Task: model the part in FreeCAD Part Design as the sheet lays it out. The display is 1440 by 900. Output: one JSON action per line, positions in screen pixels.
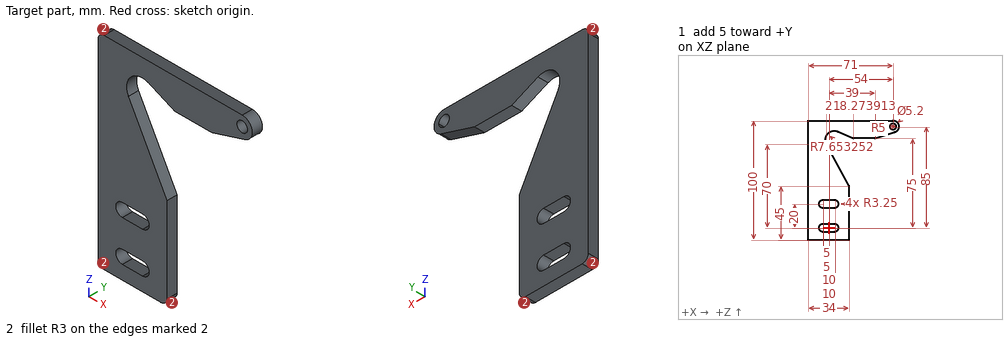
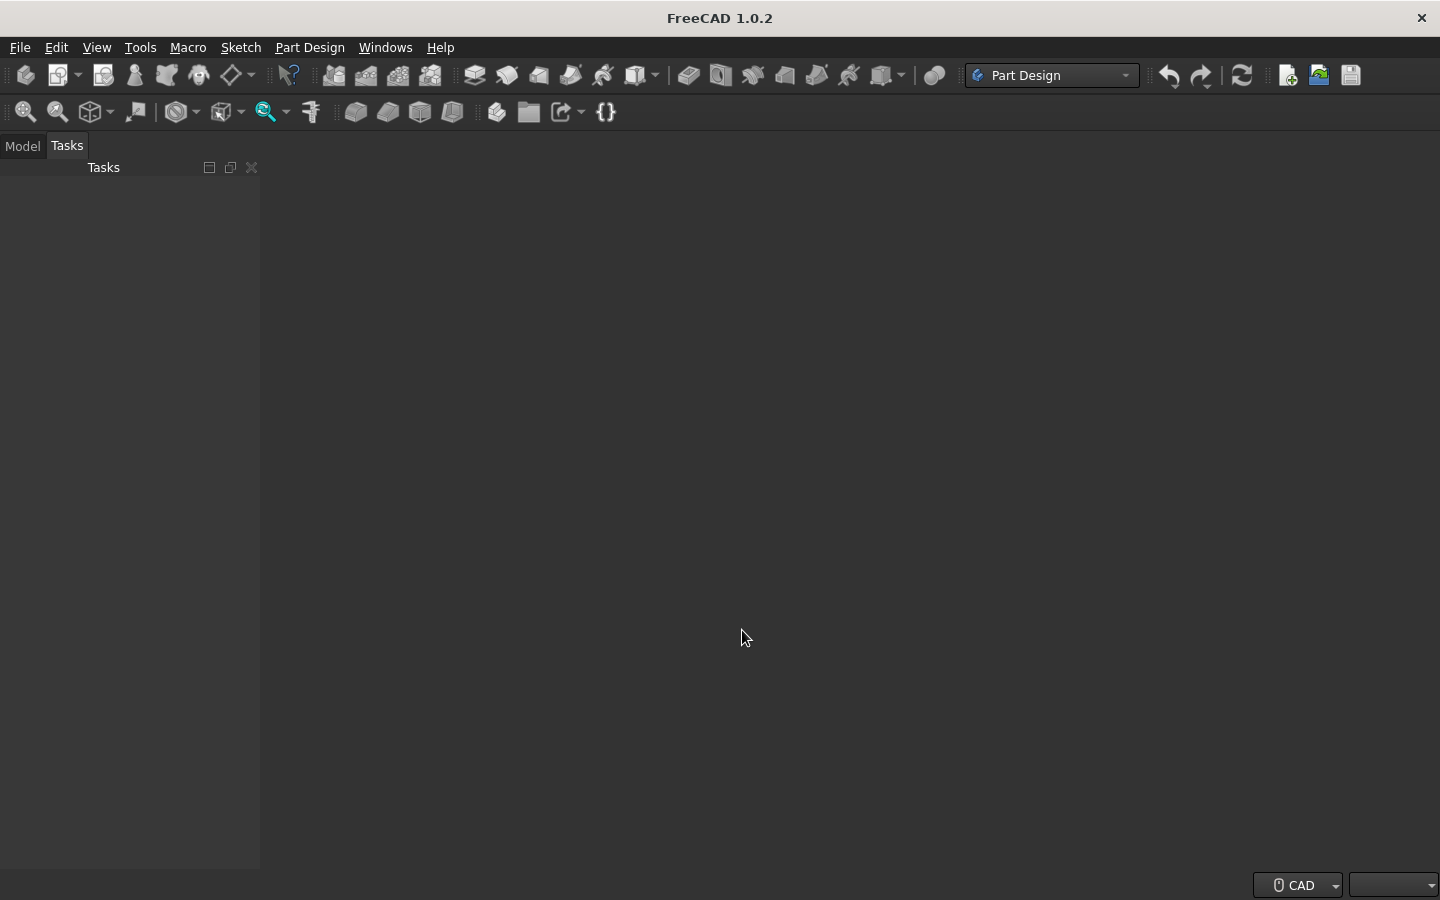
{"action": "left_click", "coordinate": [1288, 76]}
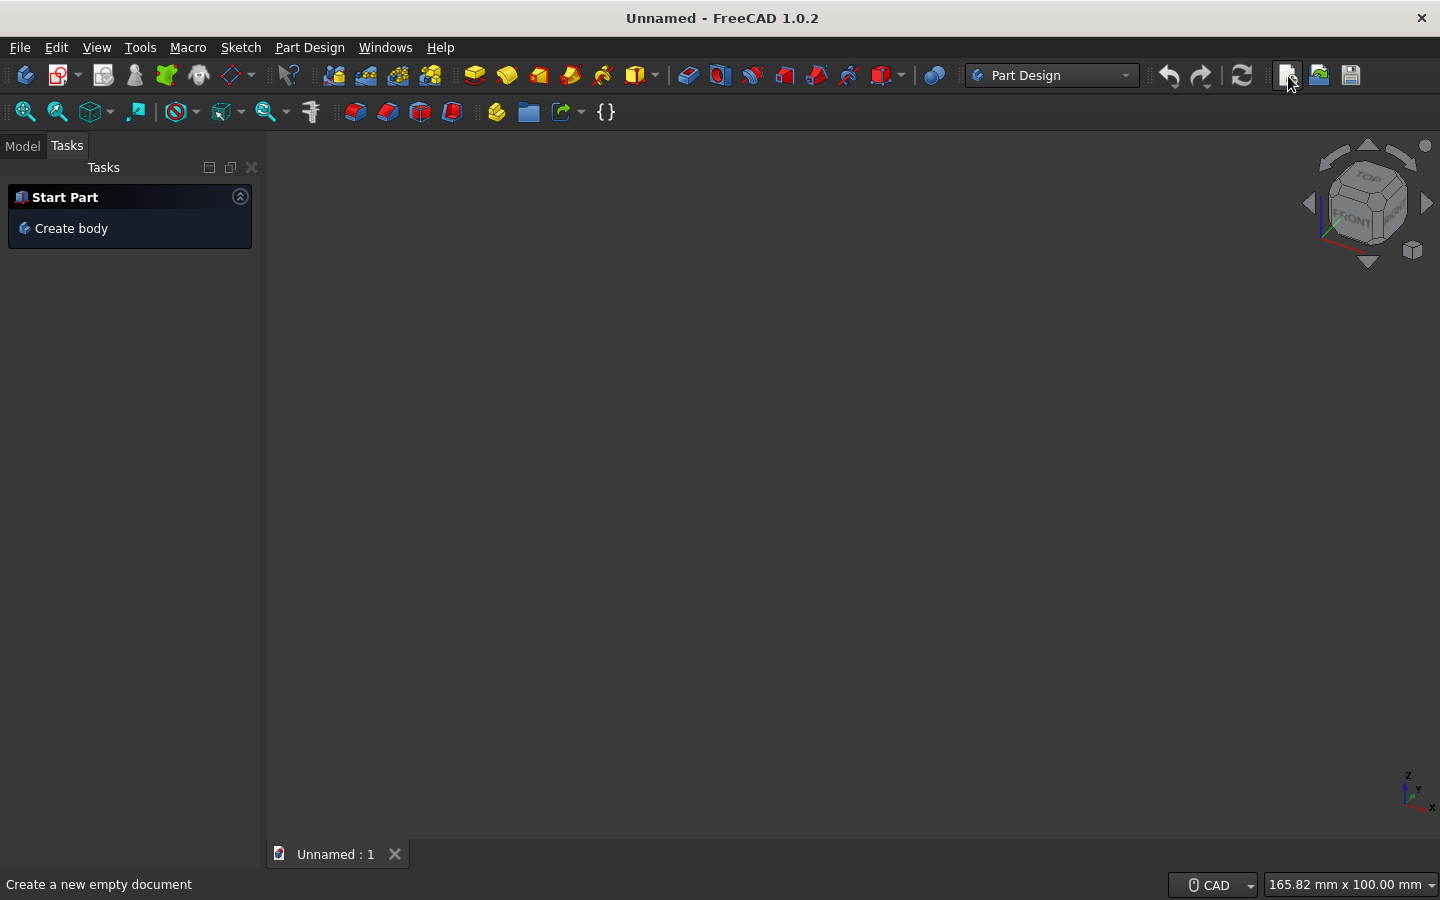
{"action": "left_click", "coordinate": [58, 76]}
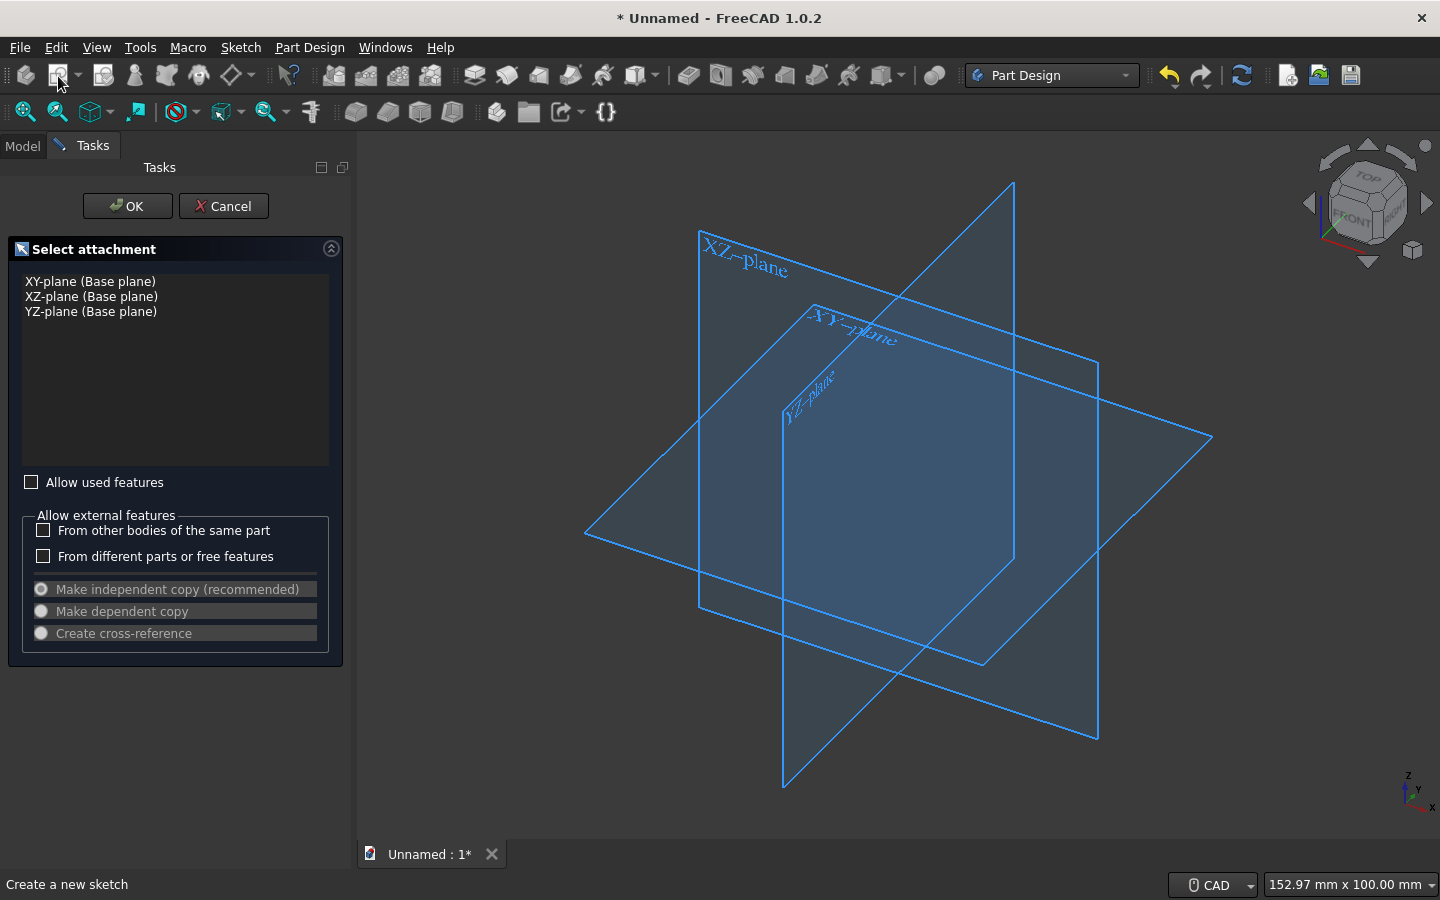
{"action": "left_click", "coordinate": [82, 296]}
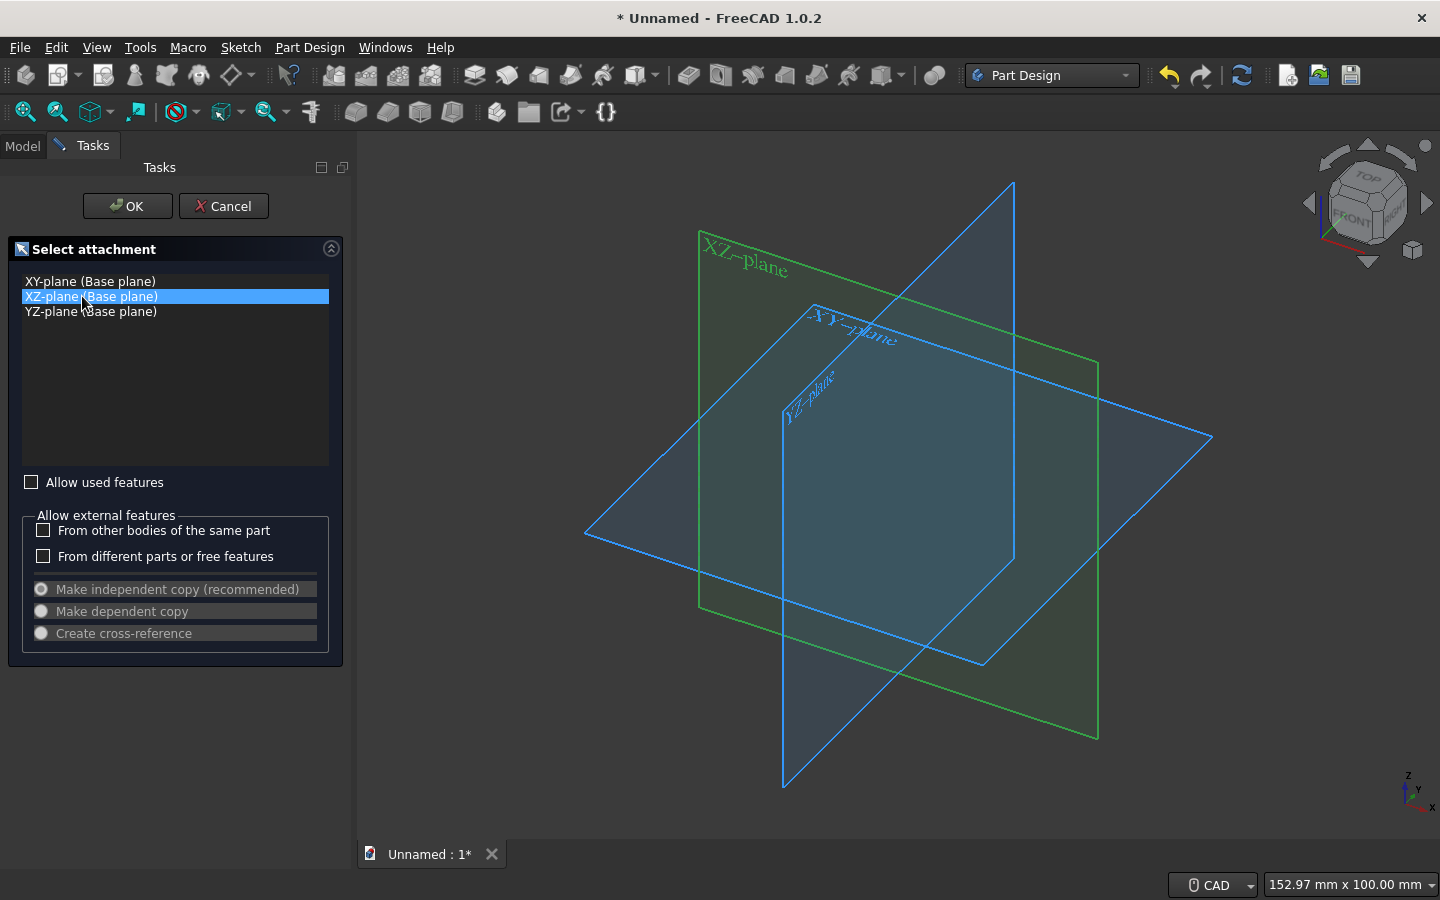
{"action": "left_click", "coordinate": [128, 206]}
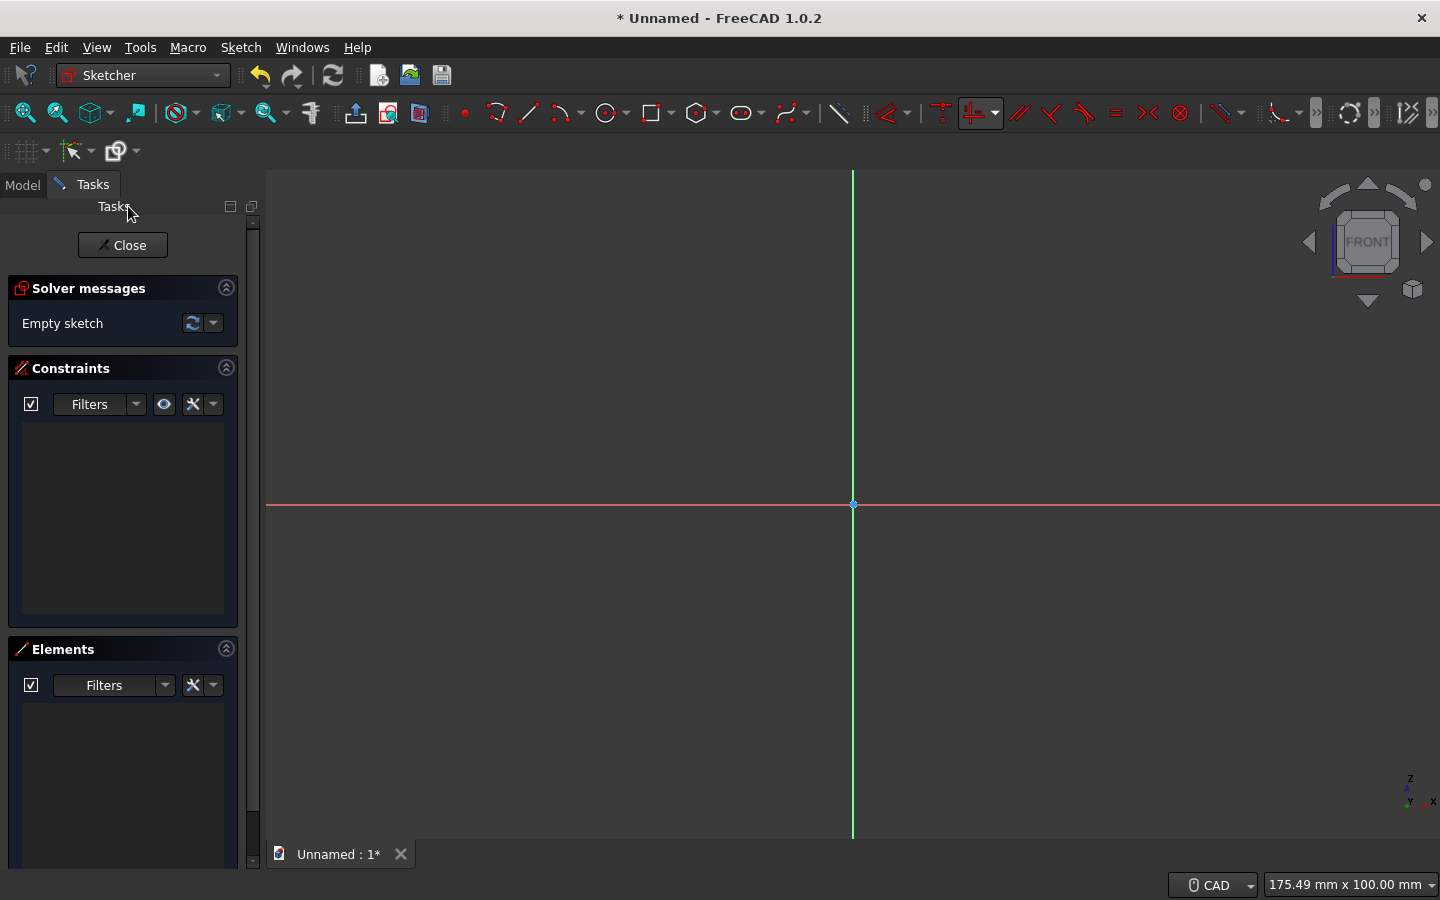
{"action": "scroll", "coordinate": [531, 811], "scroll_direction": "down", "scroll_amount": 3}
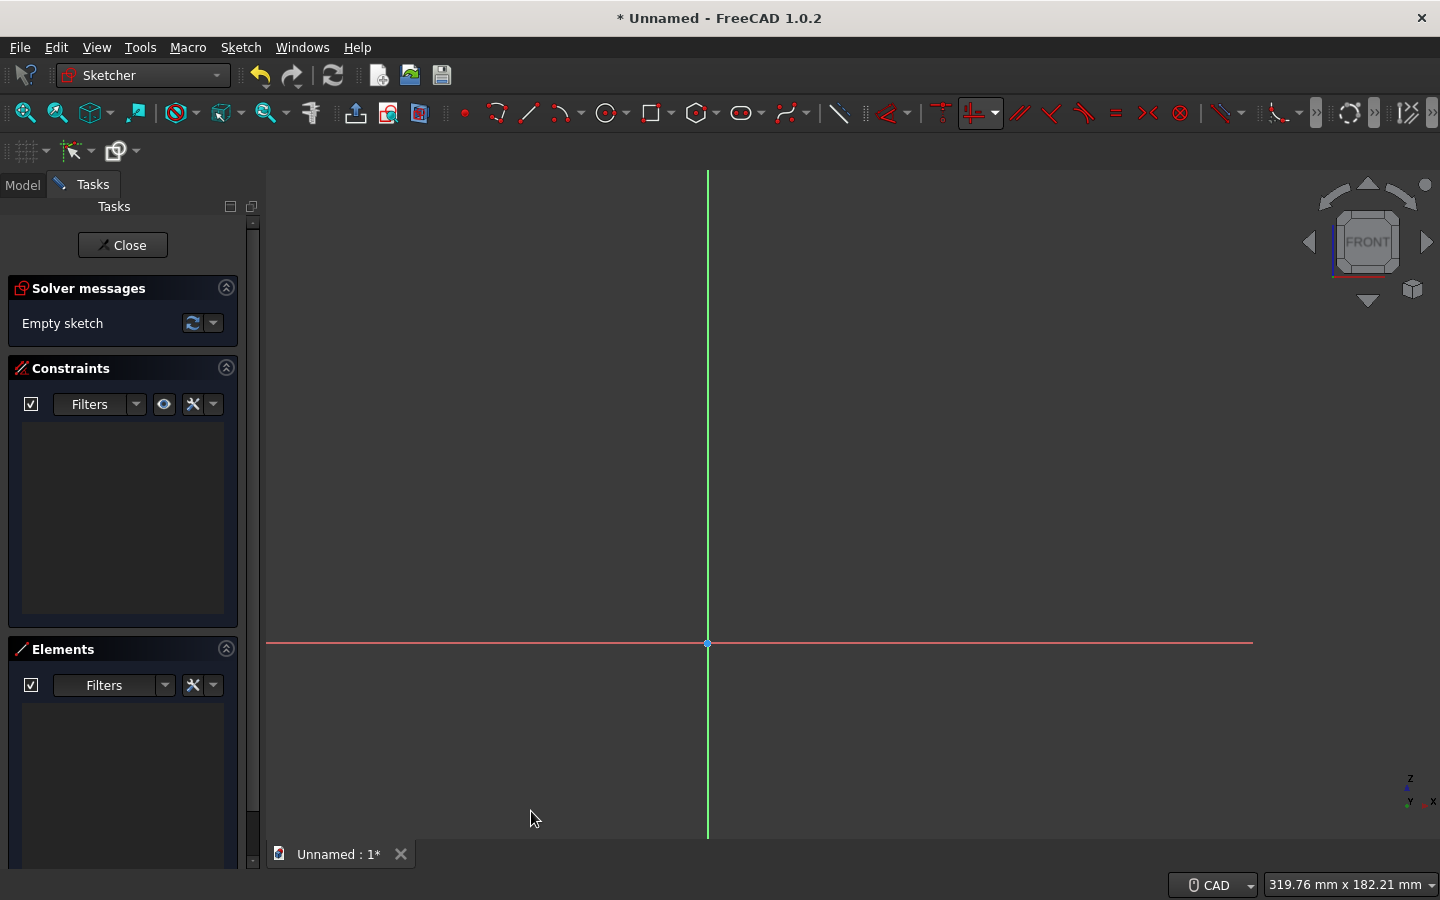
{"action": "left_click", "coordinate": [498, 114]}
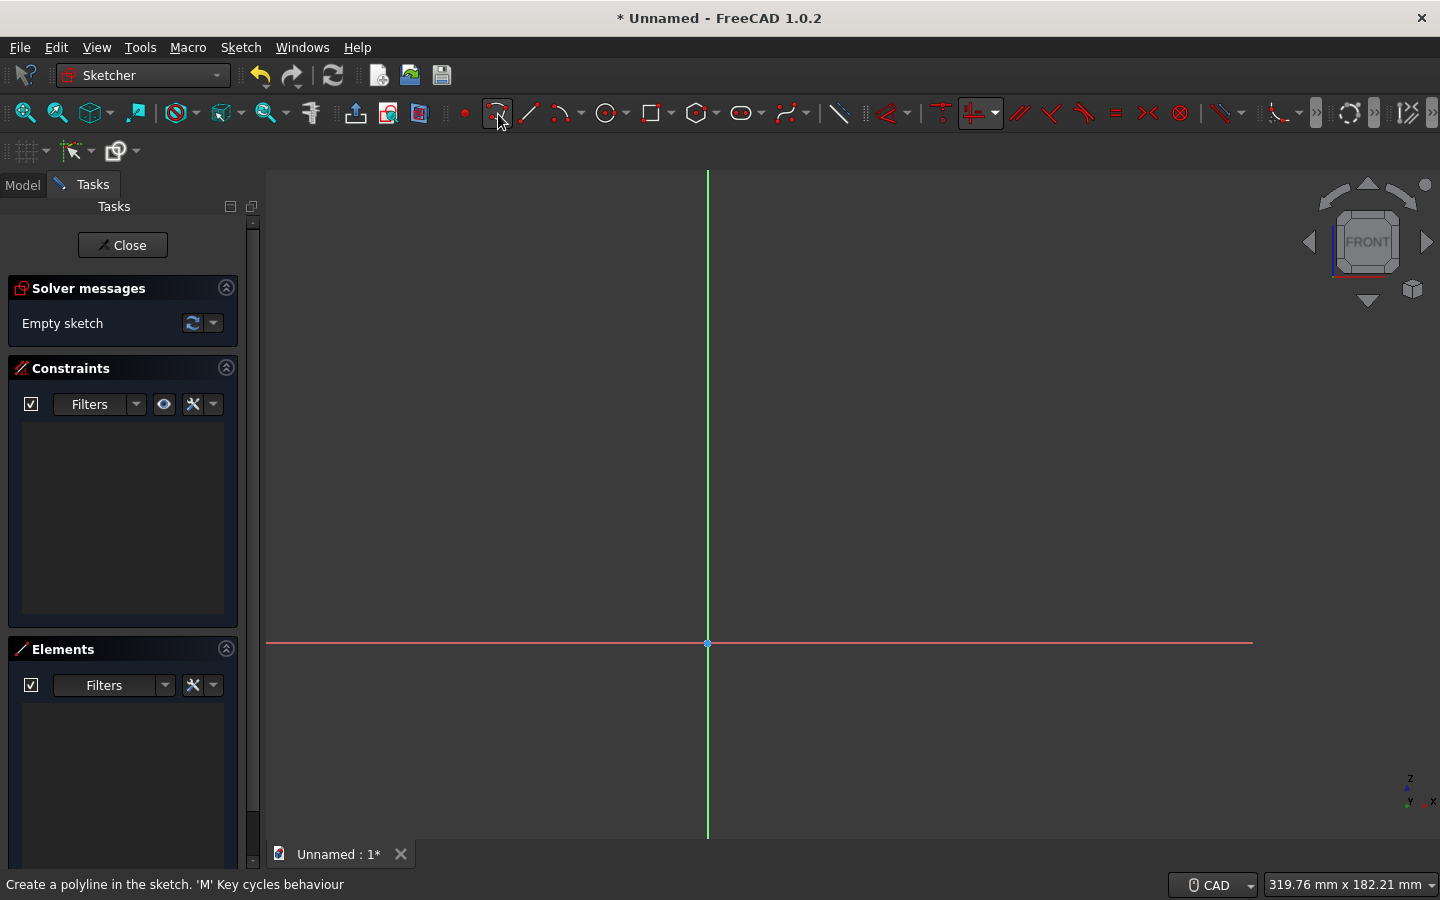
{"action": "left_click", "coordinate": [912, 349]}
{"action": "left_click", "coordinate": [851, 368]}
{"action": "left_click", "coordinate": [784, 368]}
{"action": "left_click", "coordinate": [736, 347]}
{"action": "right_click", "coordinate": [736, 347]}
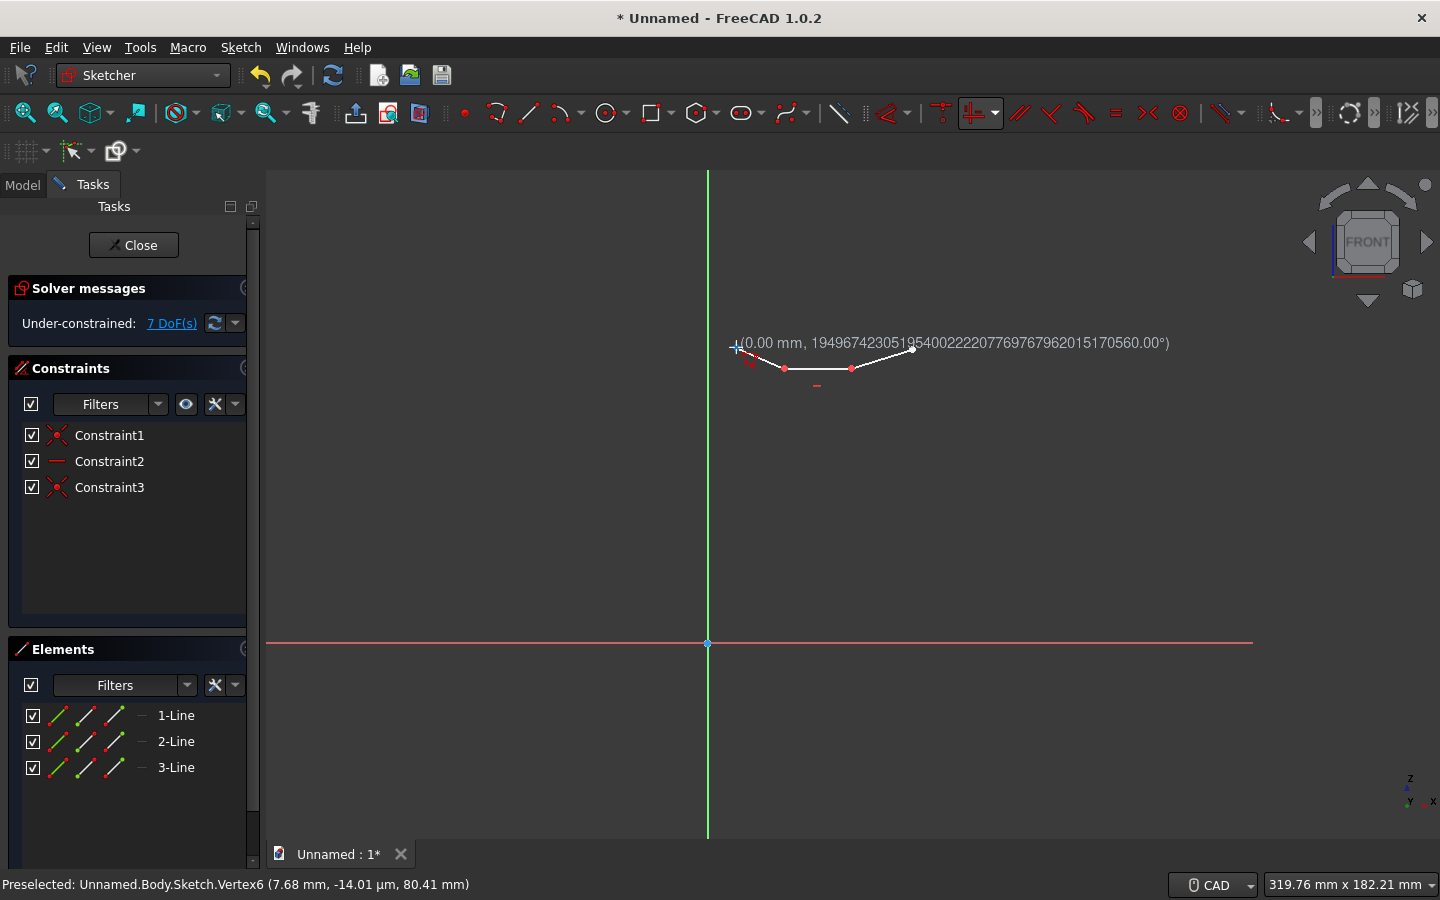
{"action": "scroll", "coordinate": [700, 386], "scroll_direction": "up", "scroll_amount": 4}